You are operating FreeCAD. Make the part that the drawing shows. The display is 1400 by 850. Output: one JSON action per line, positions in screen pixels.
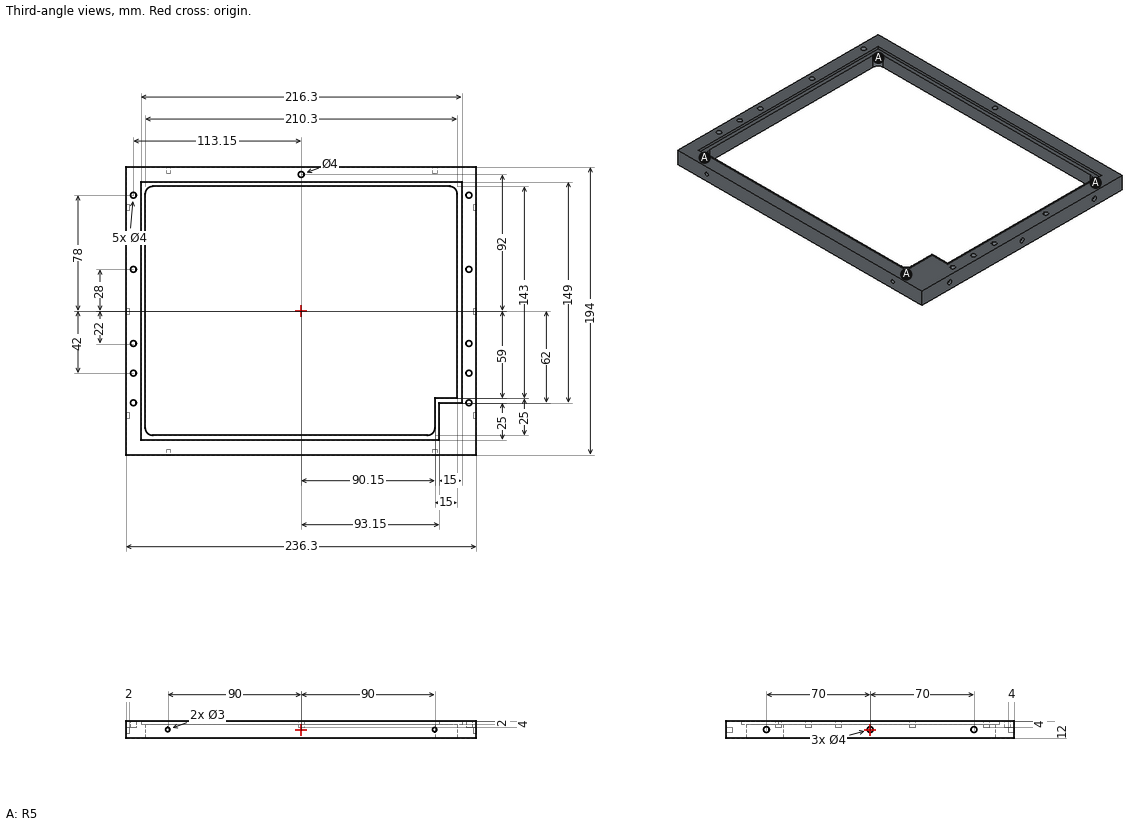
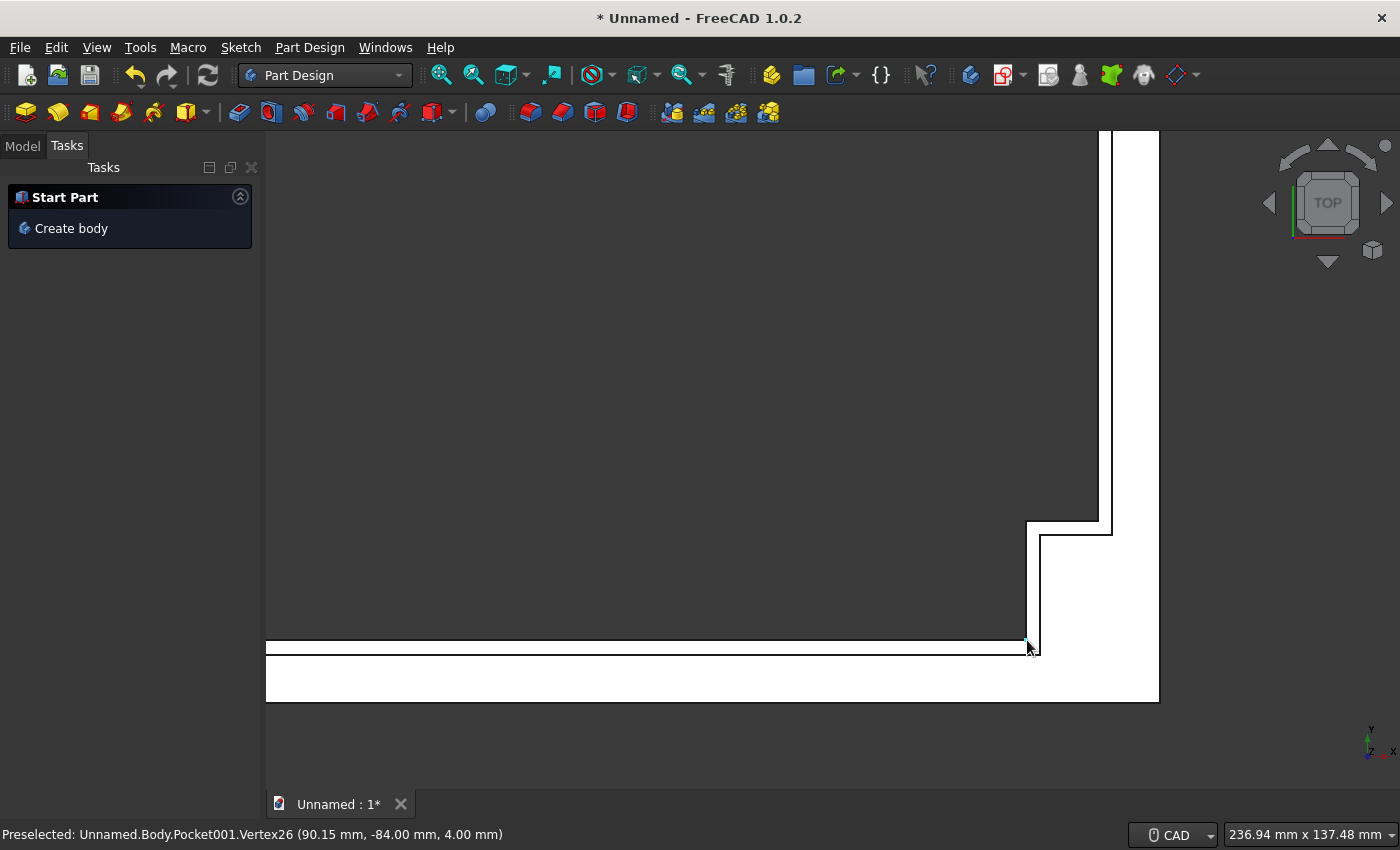
{"action": "left_click", "coordinate": [442, 76]}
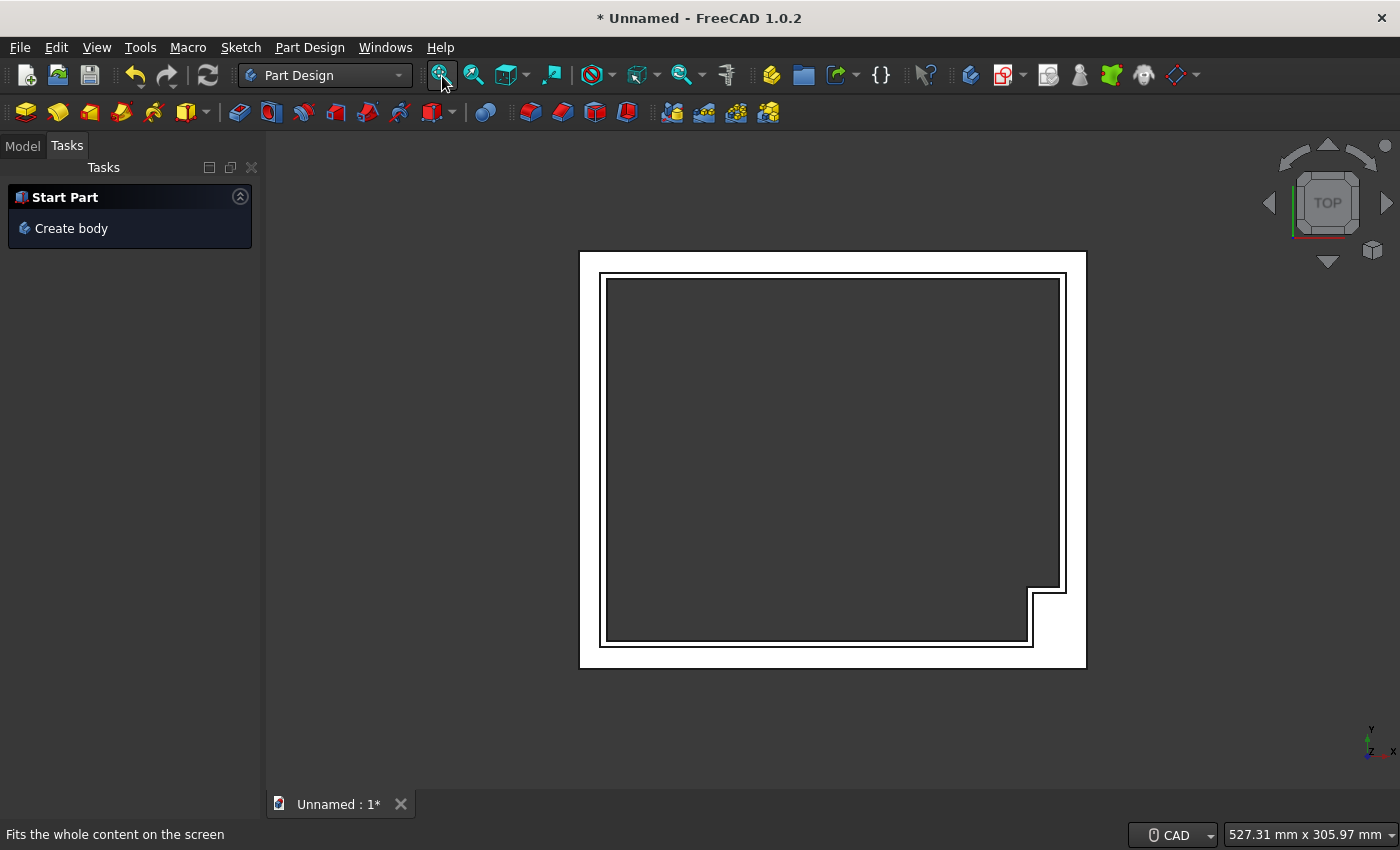
{"action": "key", "text": "1"}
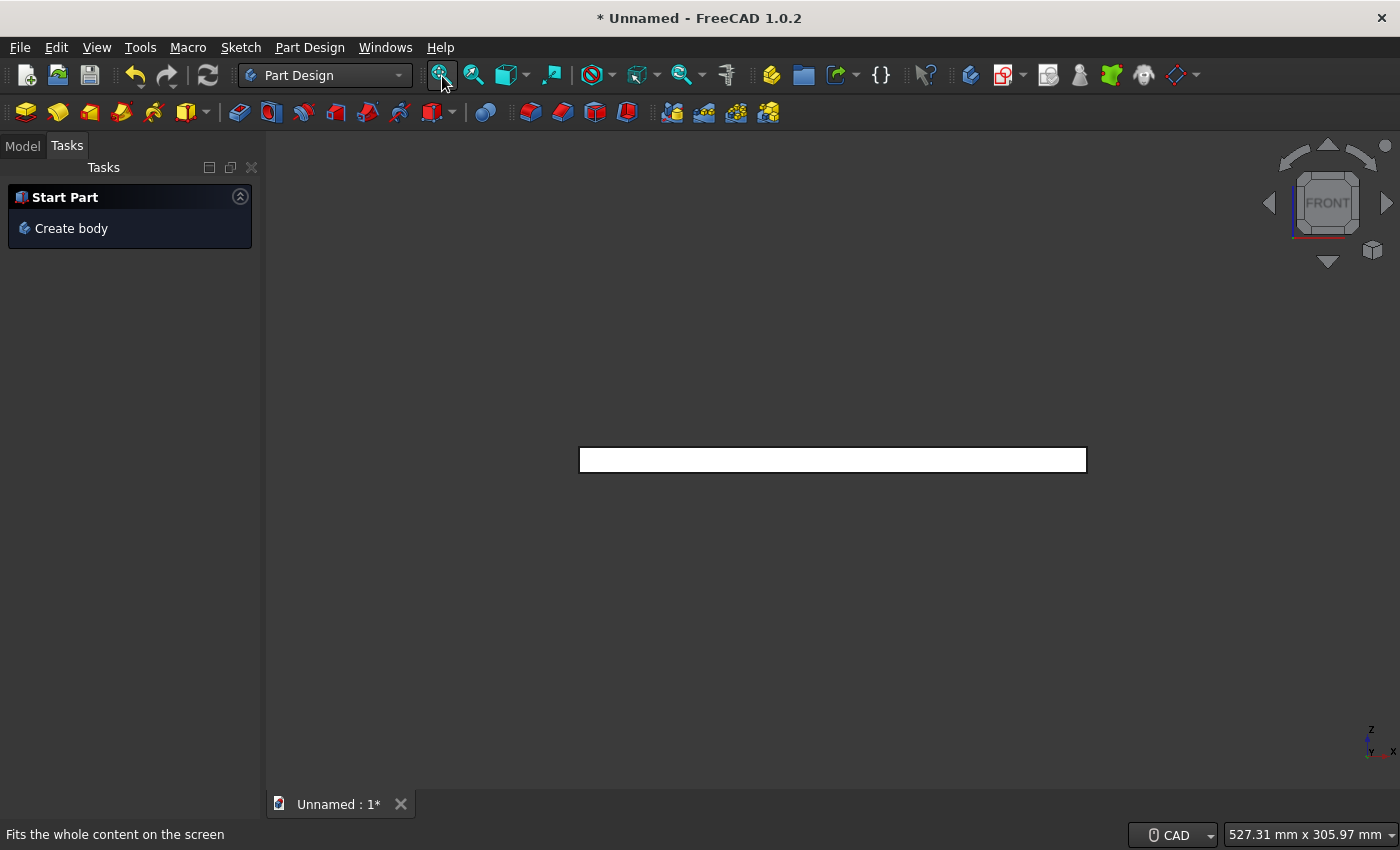
{"action": "left_click", "coordinate": [442, 76]}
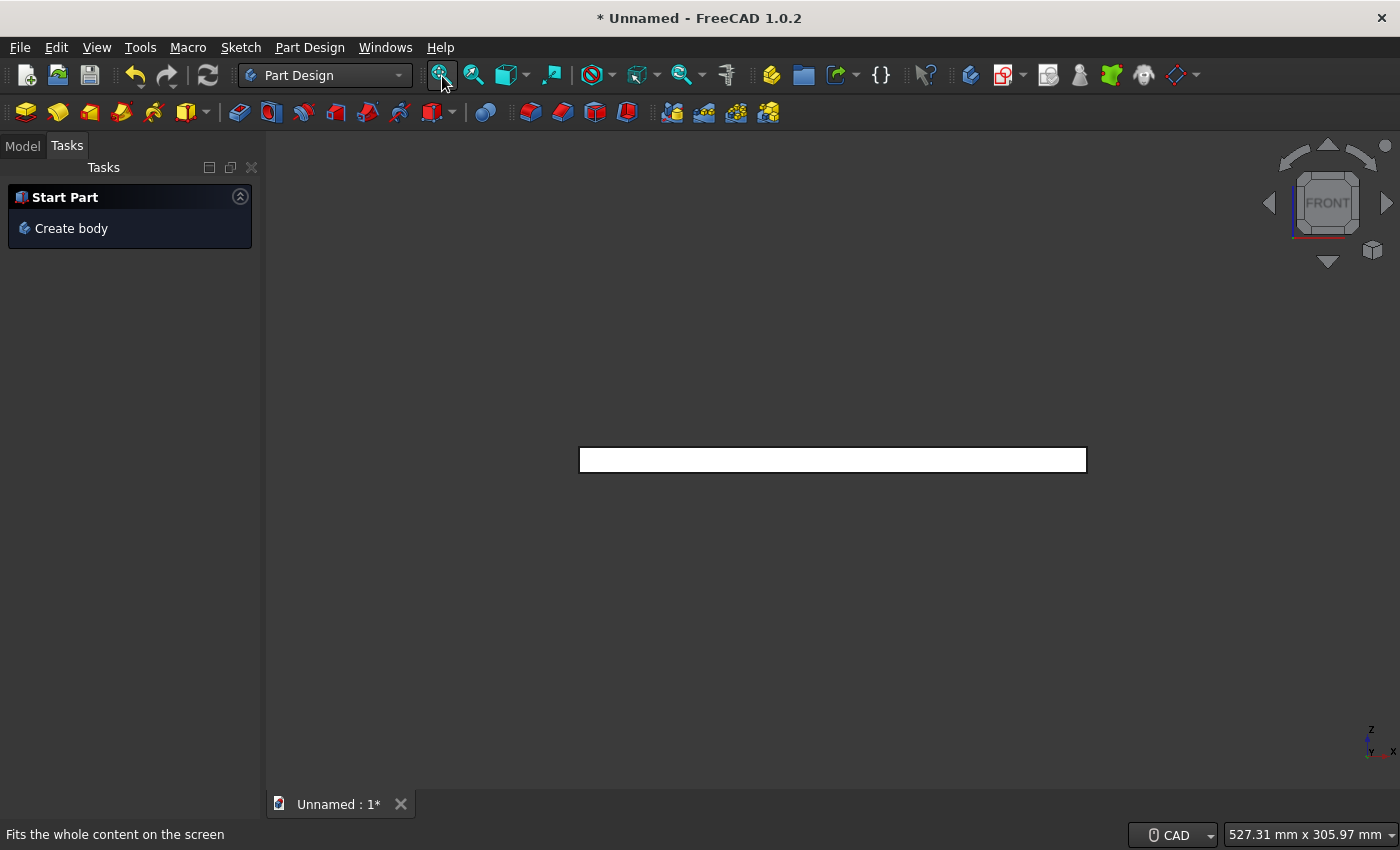
{"action": "scroll", "coordinate": [1027, 461], "scroll_direction": "up", "scroll_amount": 4}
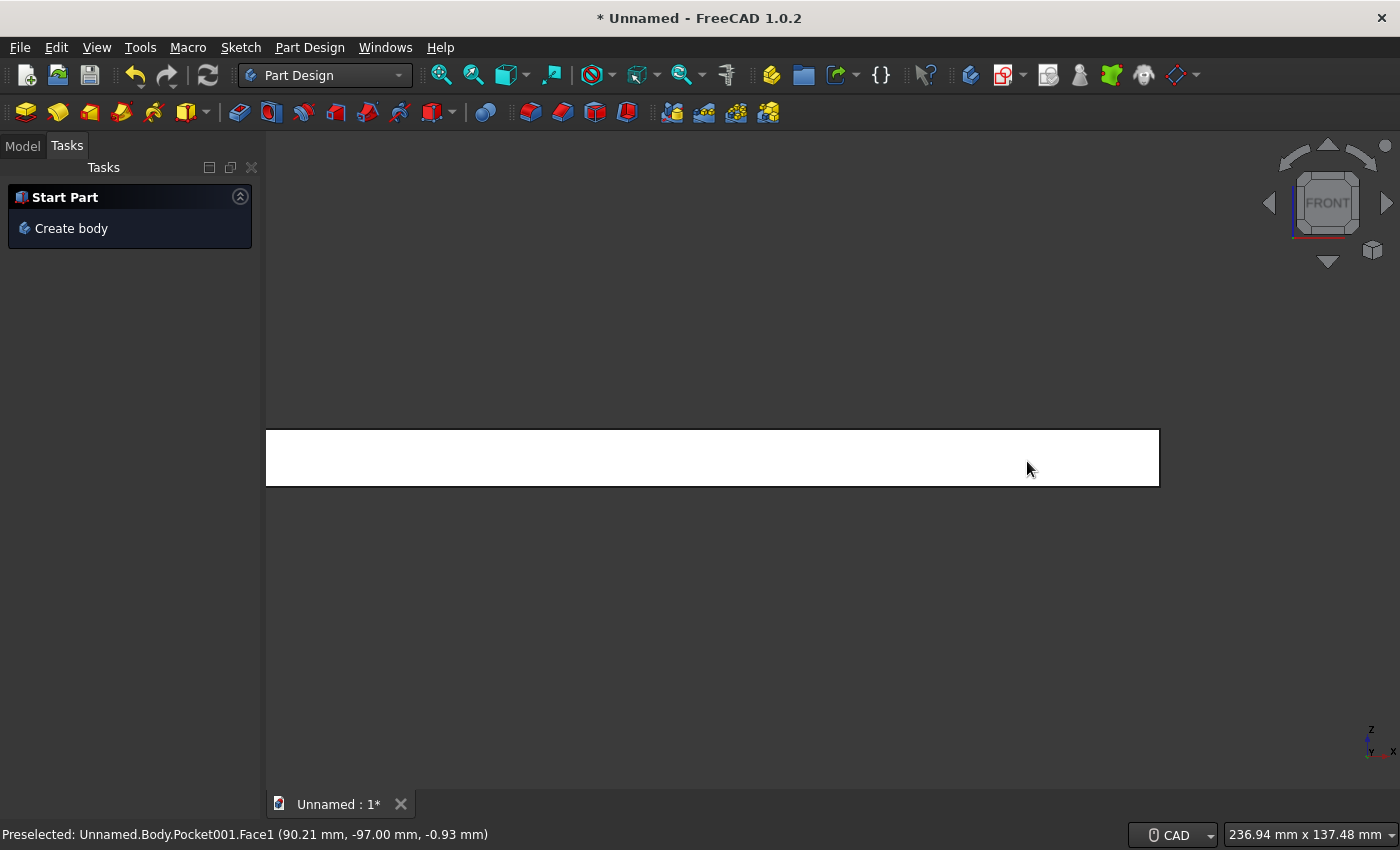
{"action": "left_click", "coordinate": [442, 76]}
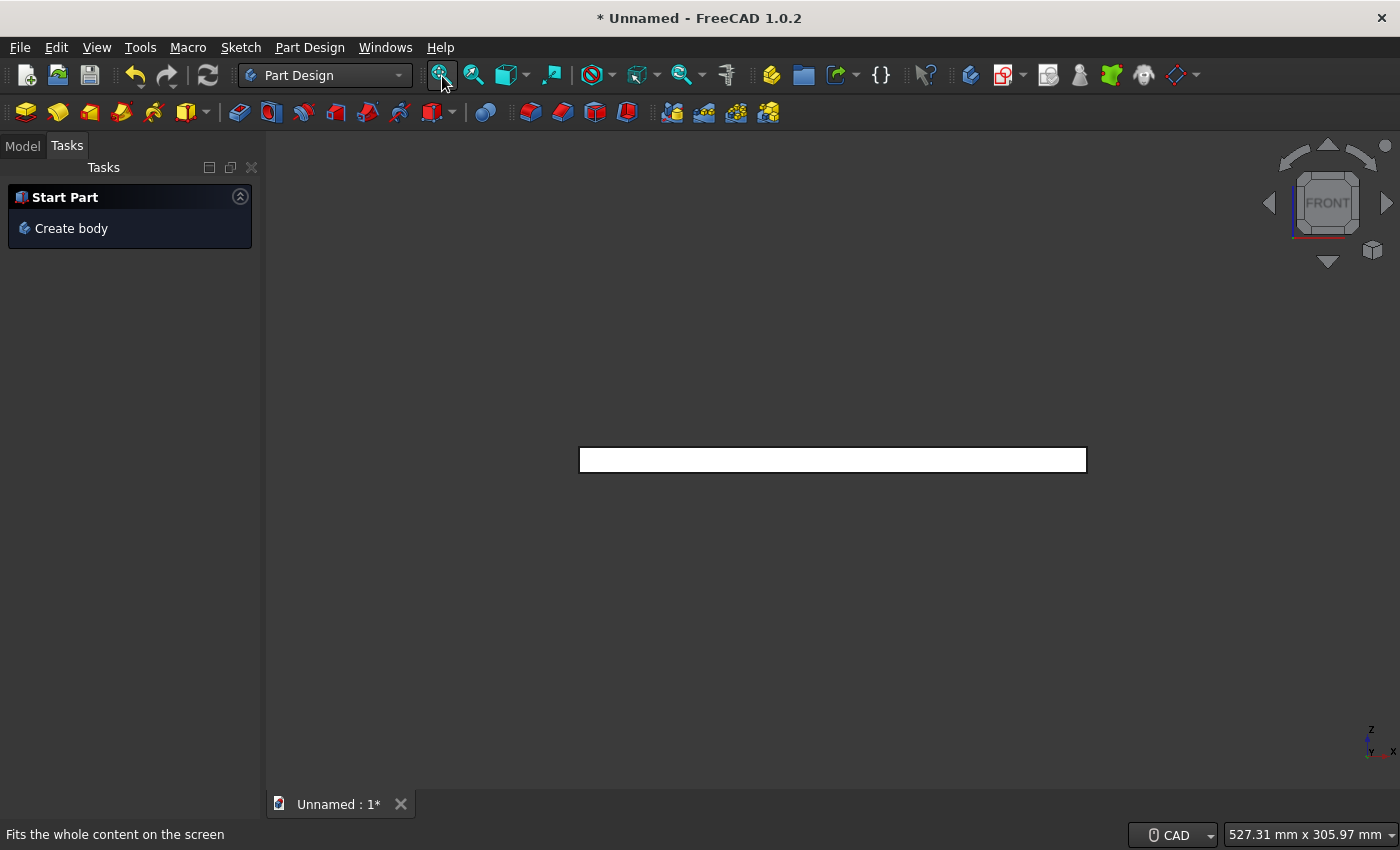
{"action": "key", "text": "3"}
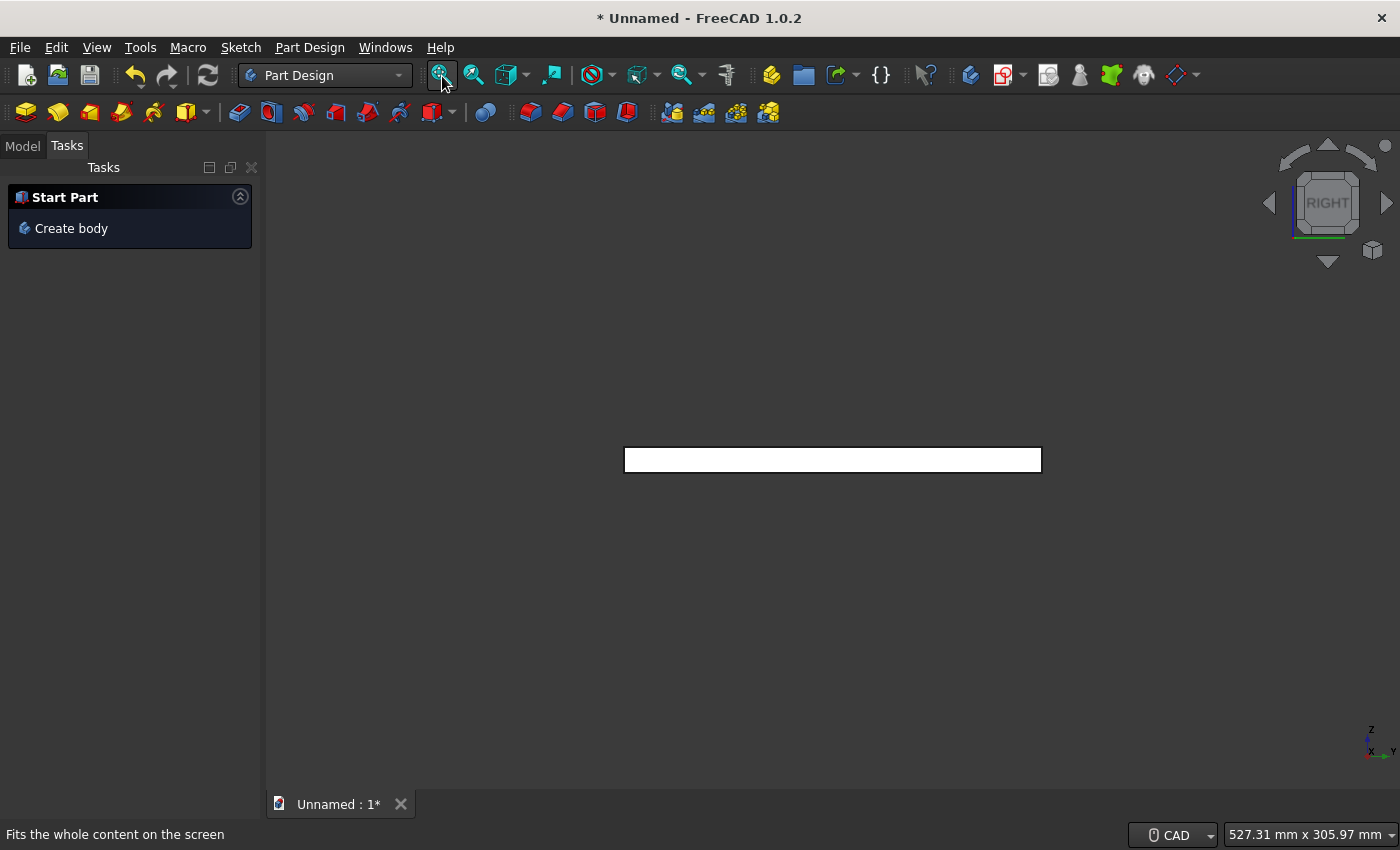
{"action": "left_click", "coordinate": [442, 76]}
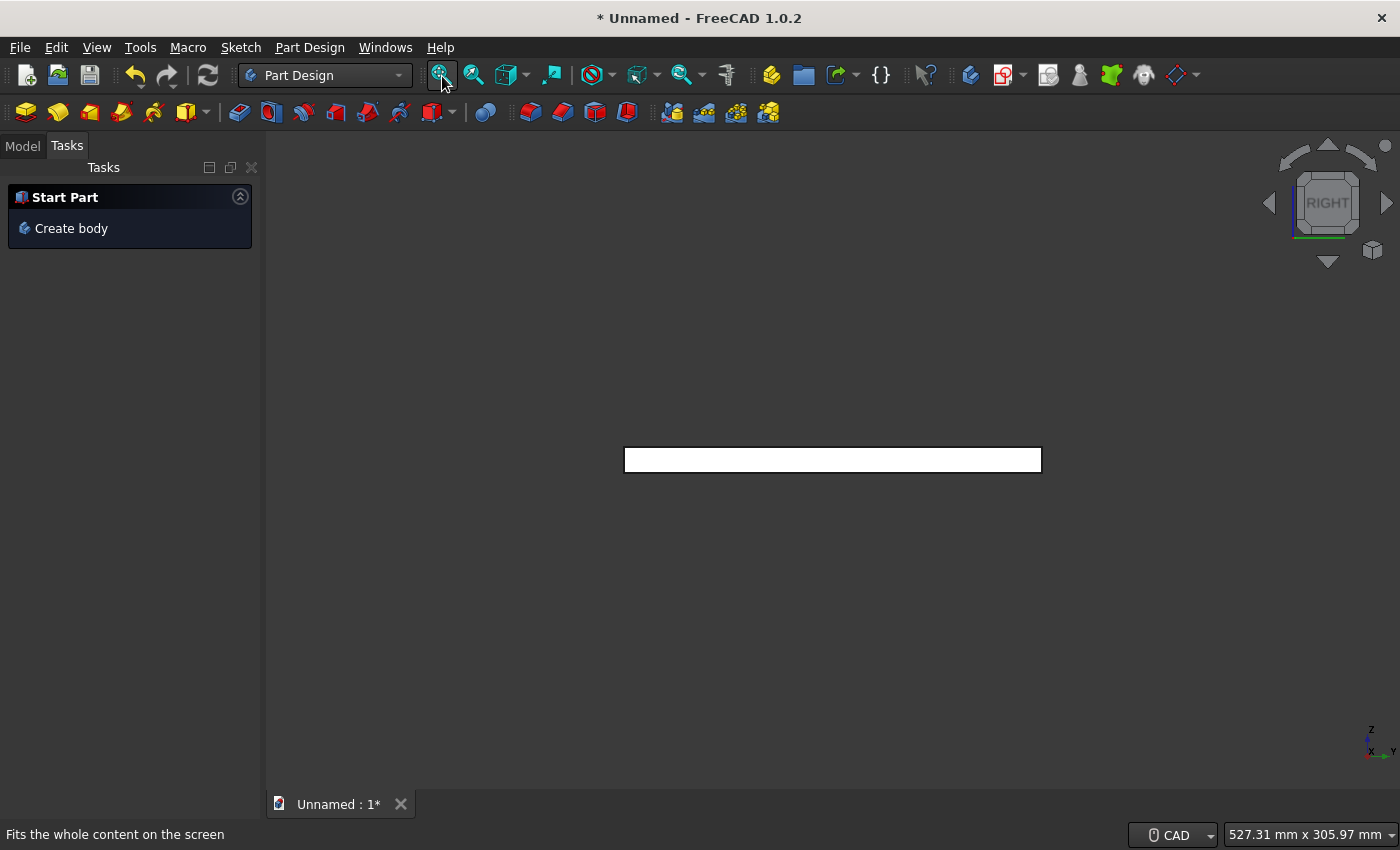
{"action": "scroll", "coordinate": [652, 461], "scroll_direction": "up", "scroll_amount": 4}